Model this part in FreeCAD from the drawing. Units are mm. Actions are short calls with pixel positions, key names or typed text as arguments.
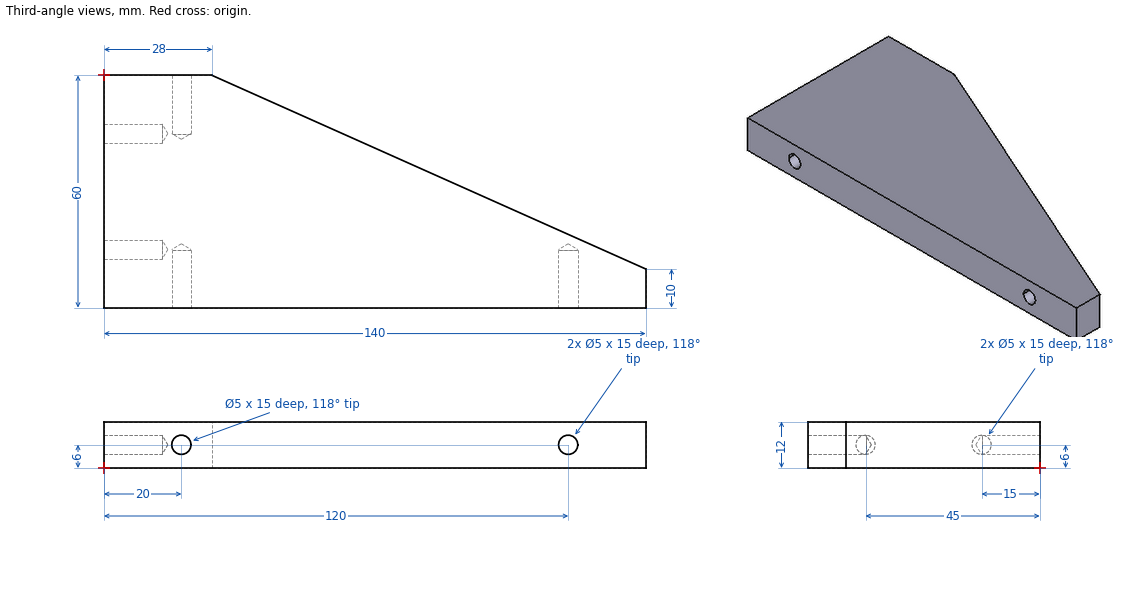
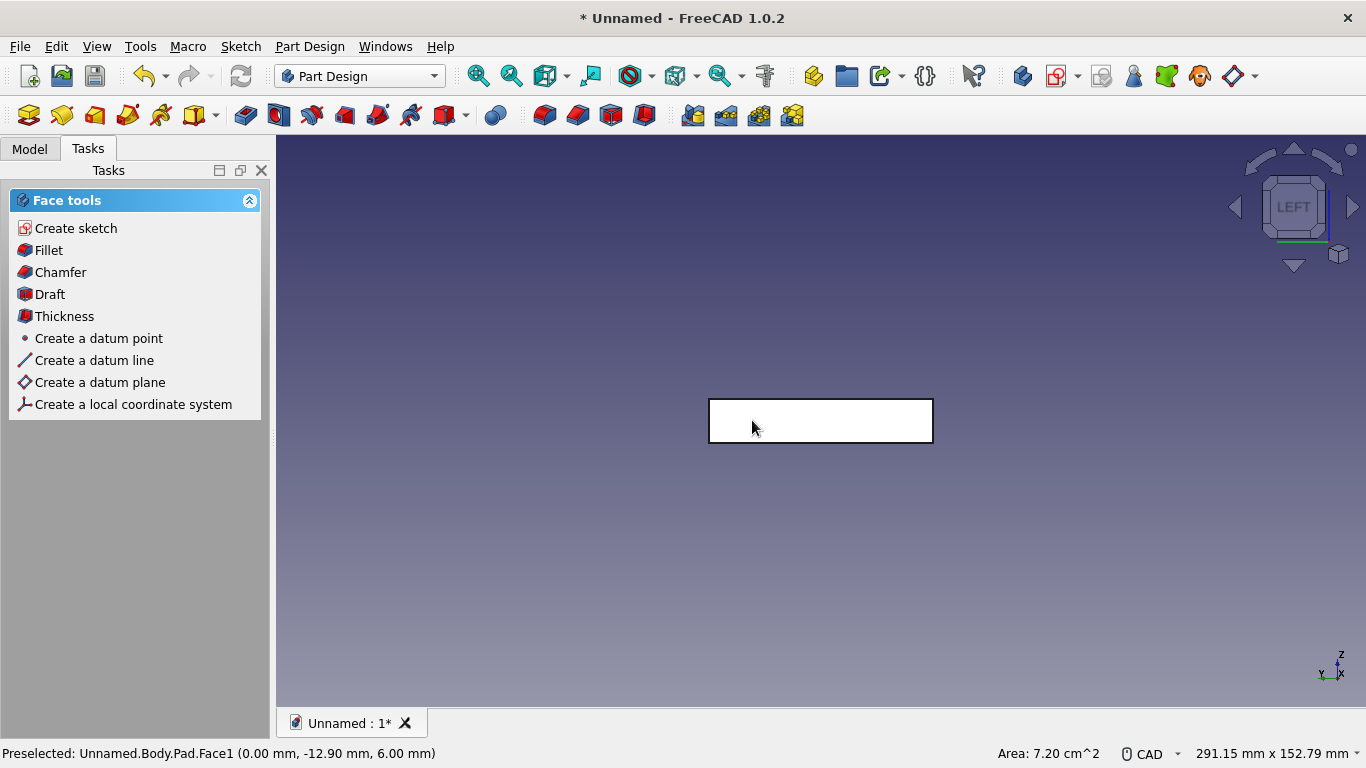
click(1056, 76)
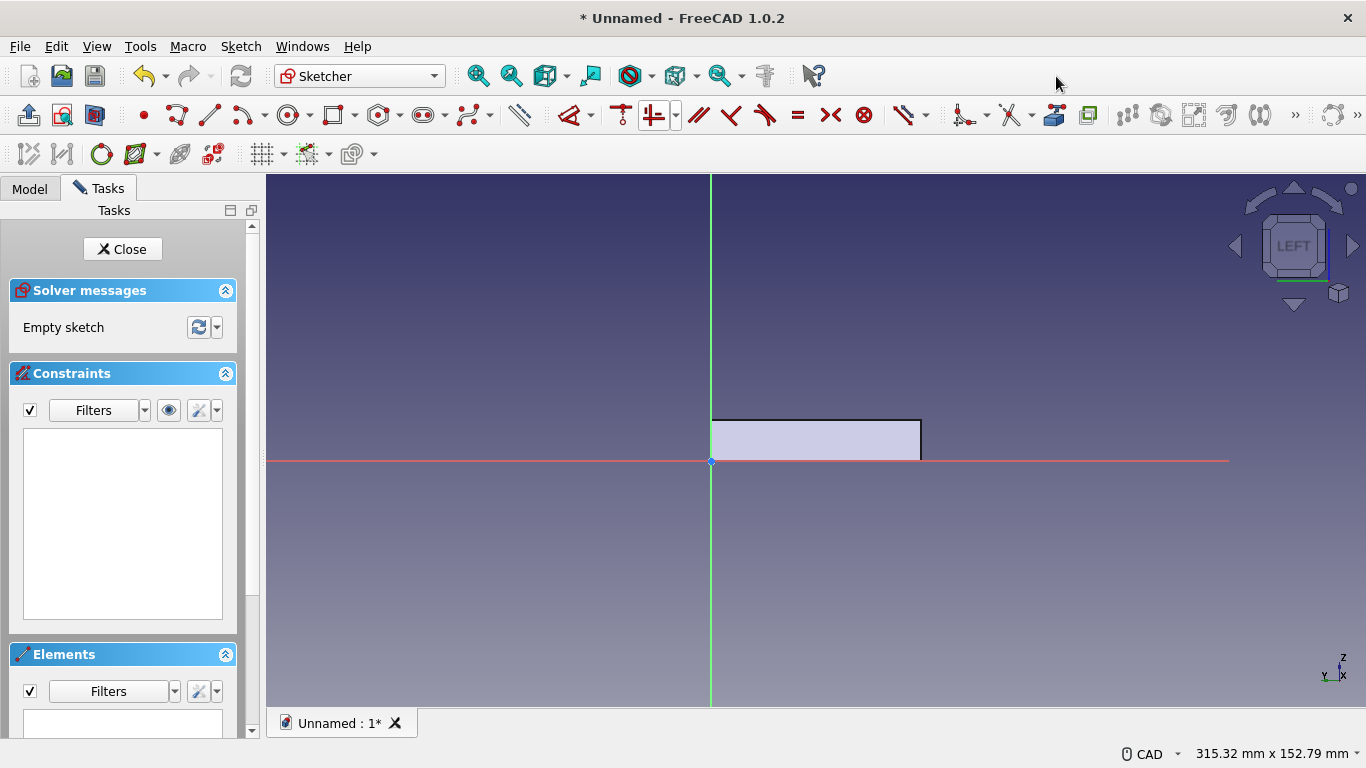
scroll(809, 449, up, 7)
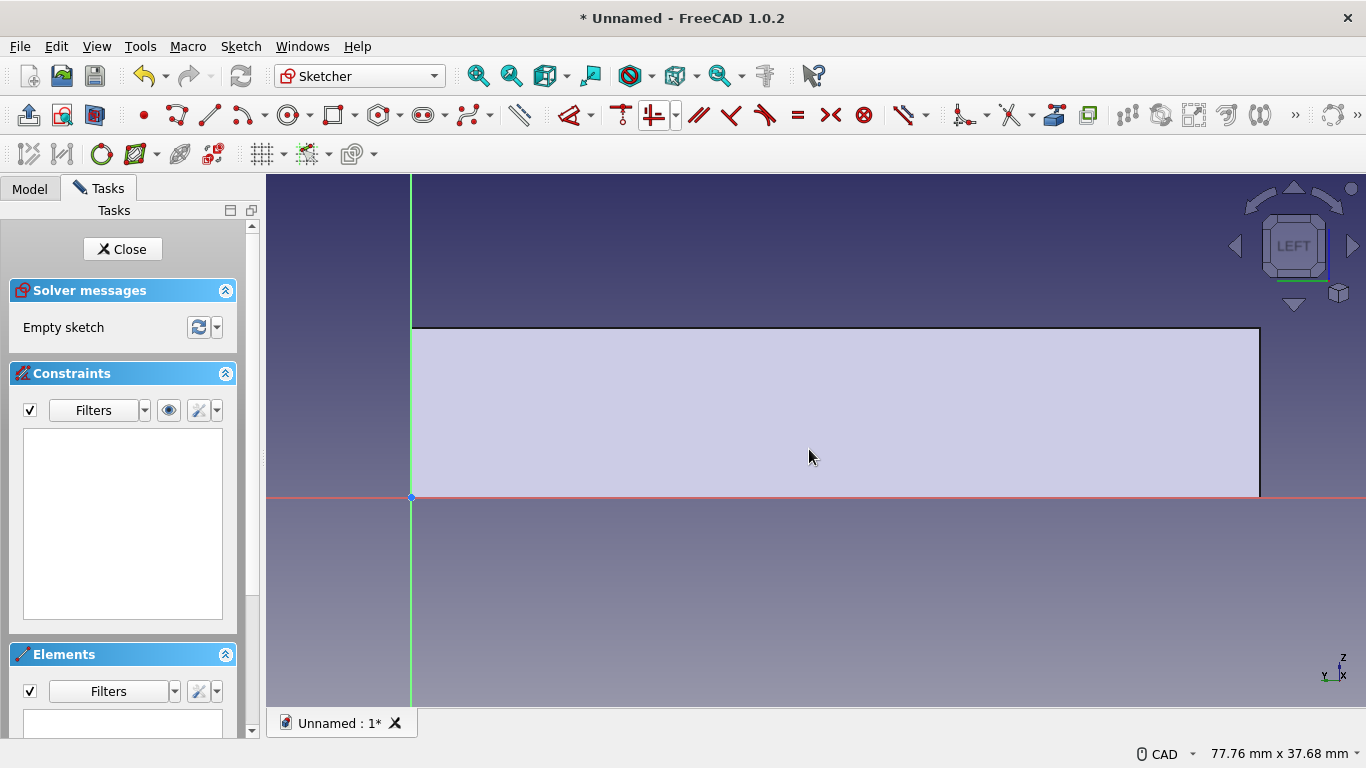
key(g)
key(c)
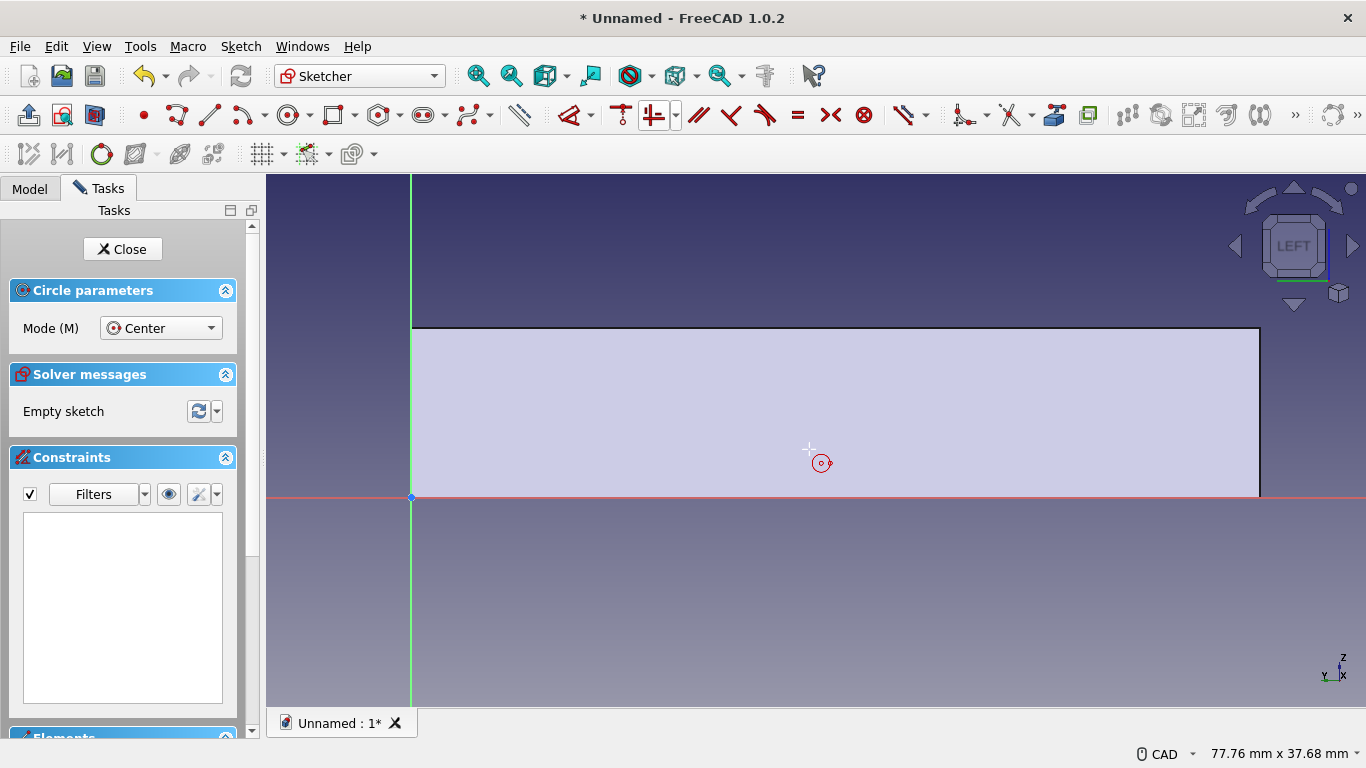
click(624, 413)
move(649, 388)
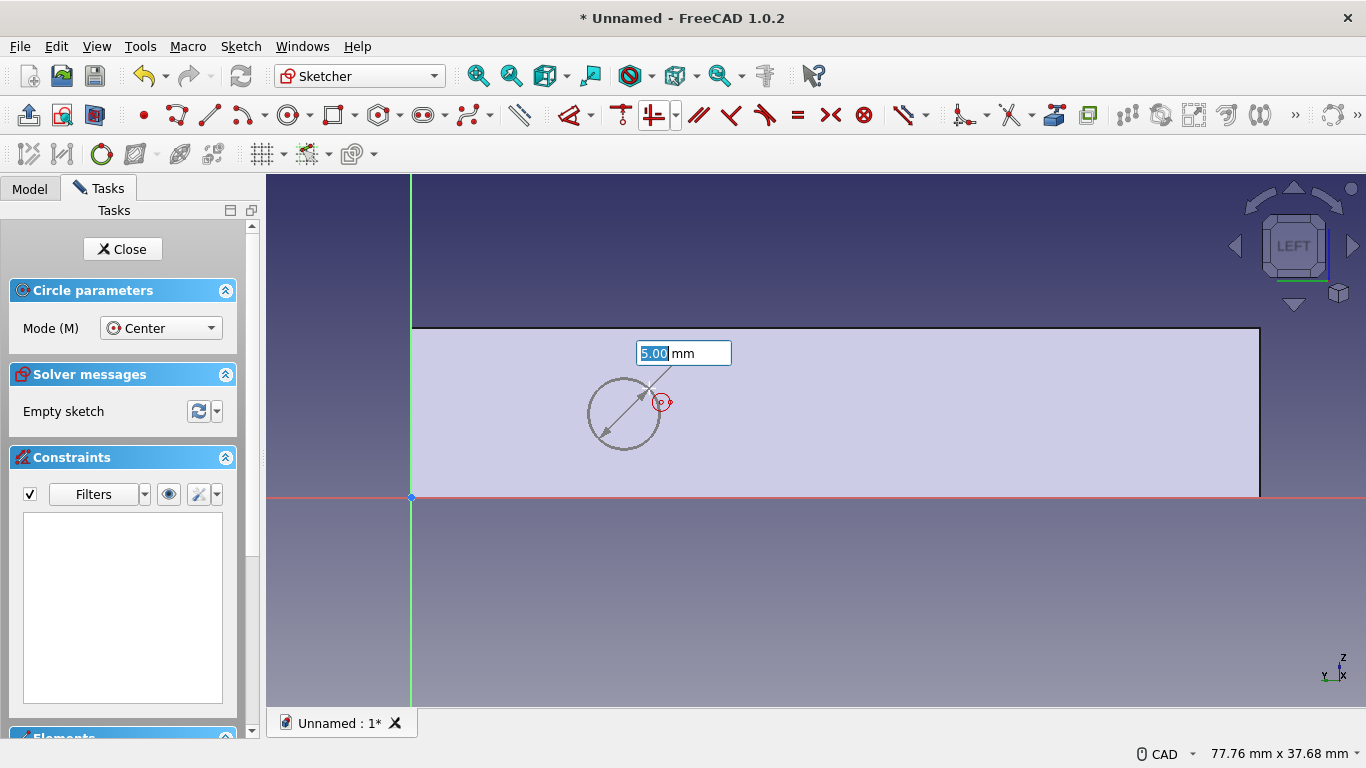
text(5)
key(Return)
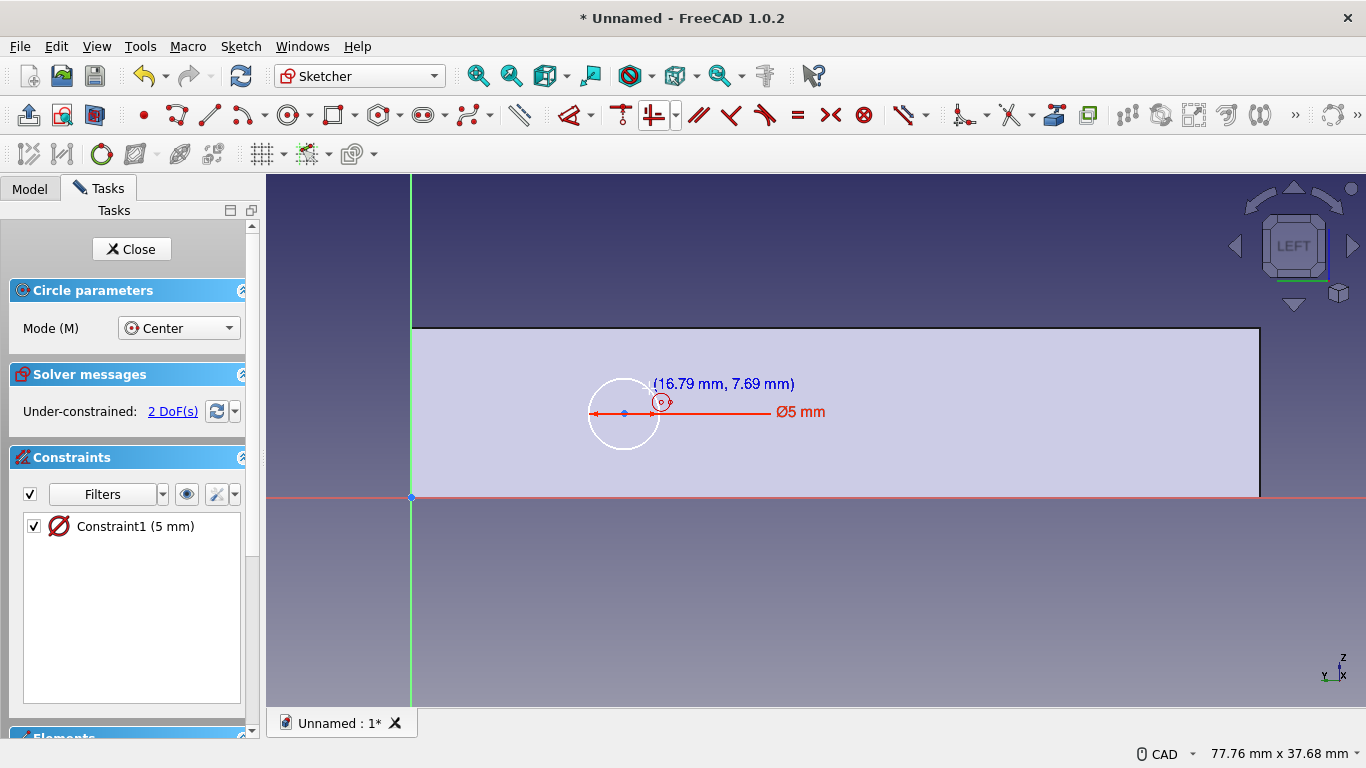
click(1048, 413)
move(1073, 388)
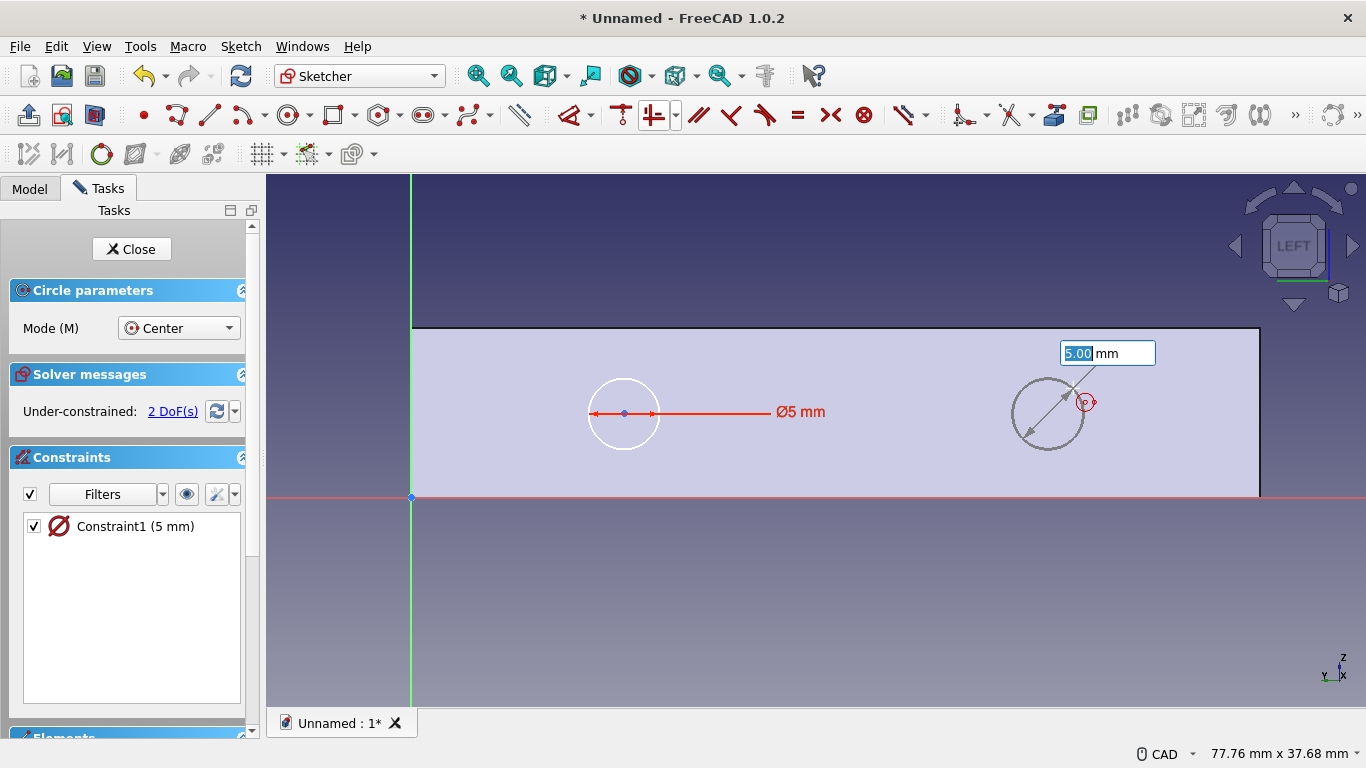
text(5)
key(Return)
key(Escape)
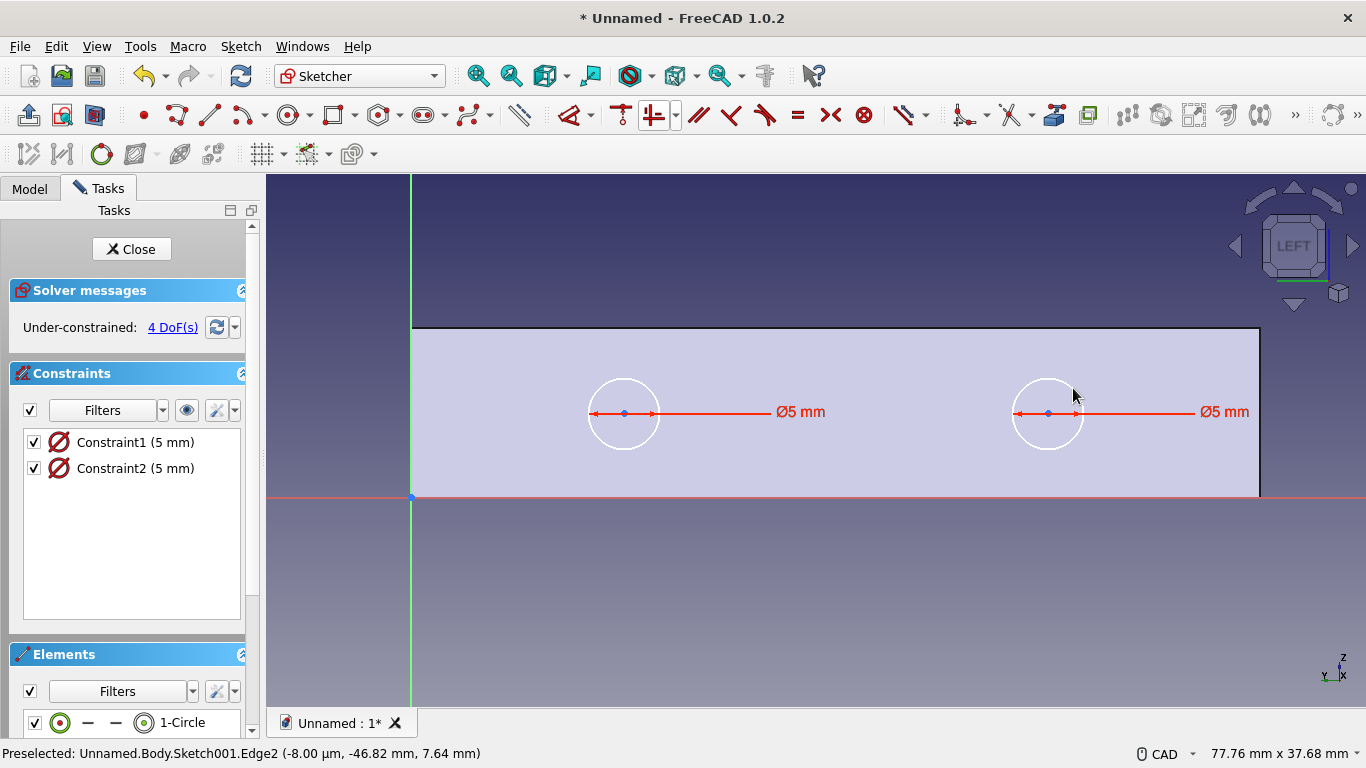
click(624, 414)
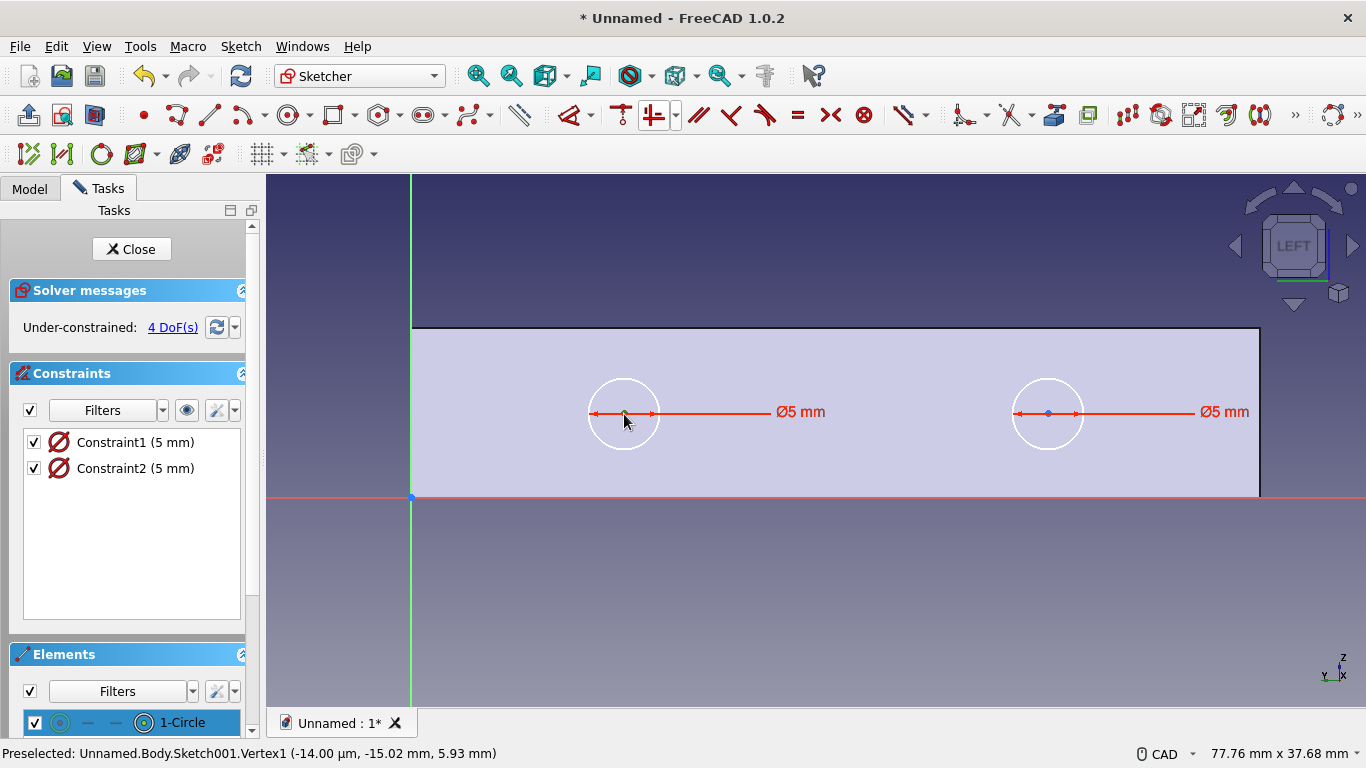
click(1048, 414)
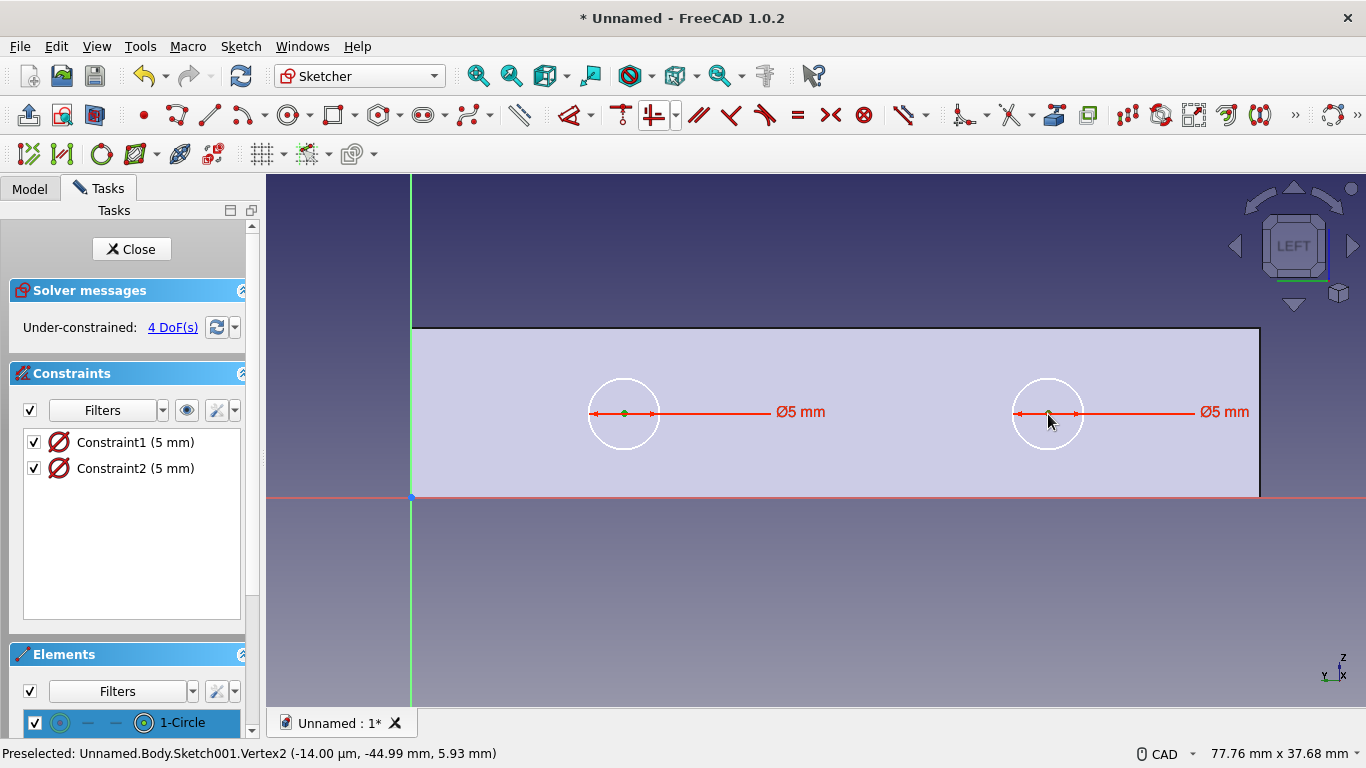
key(h)